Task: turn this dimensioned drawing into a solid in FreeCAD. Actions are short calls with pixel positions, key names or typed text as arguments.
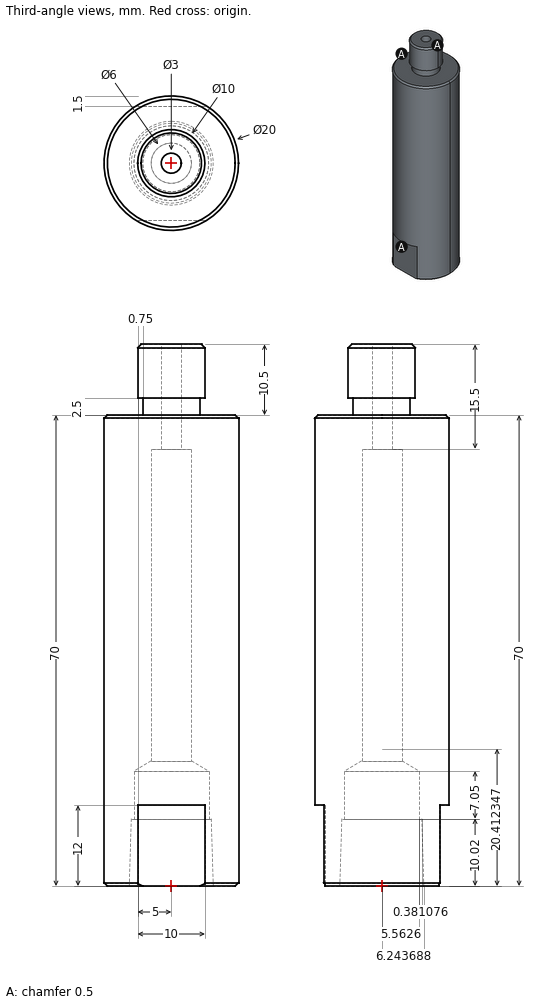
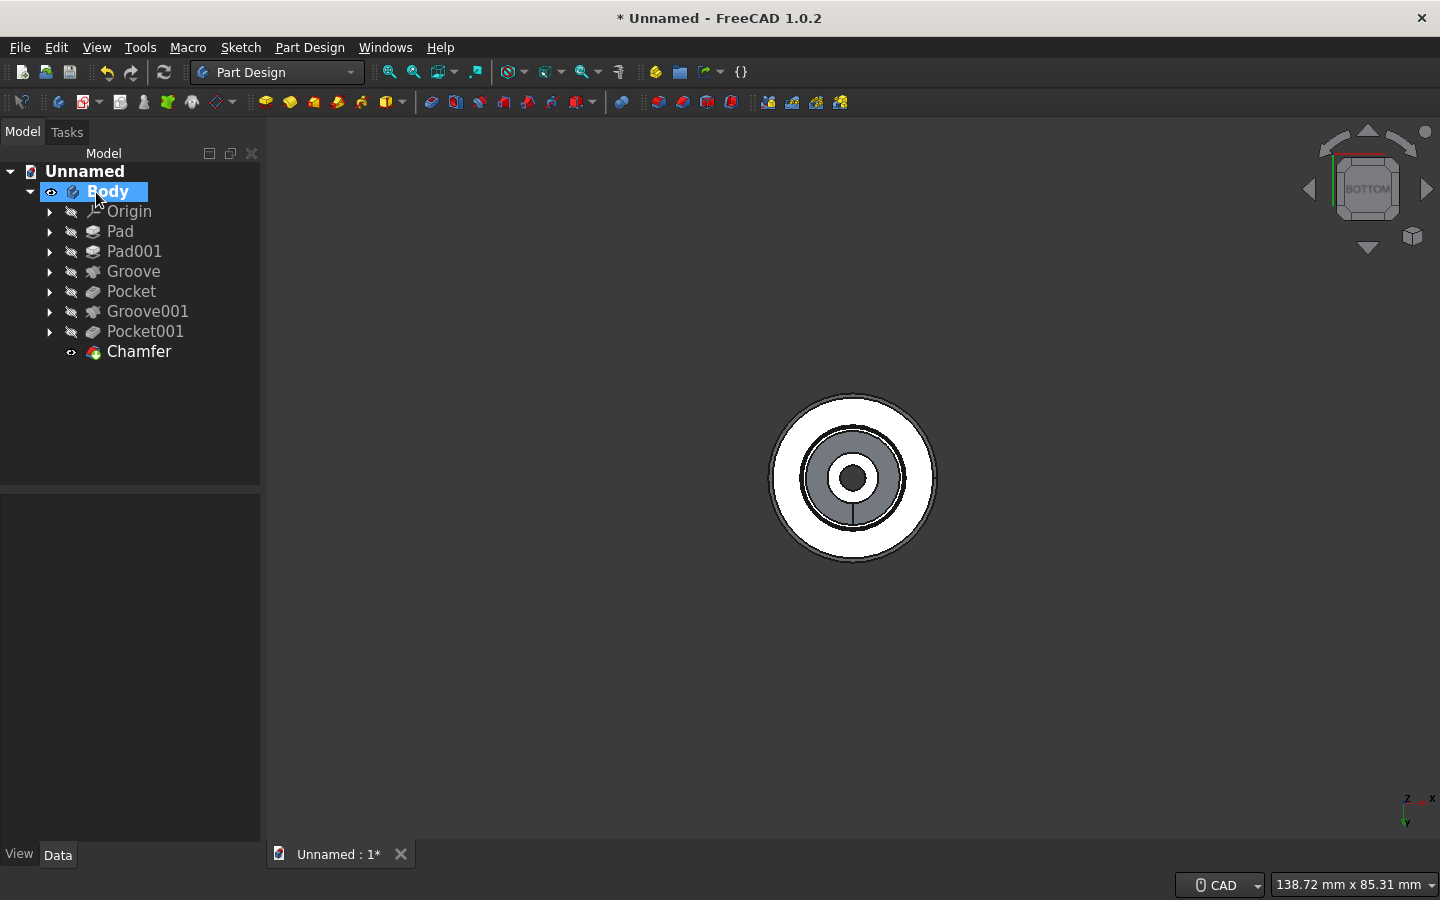
click(390, 72)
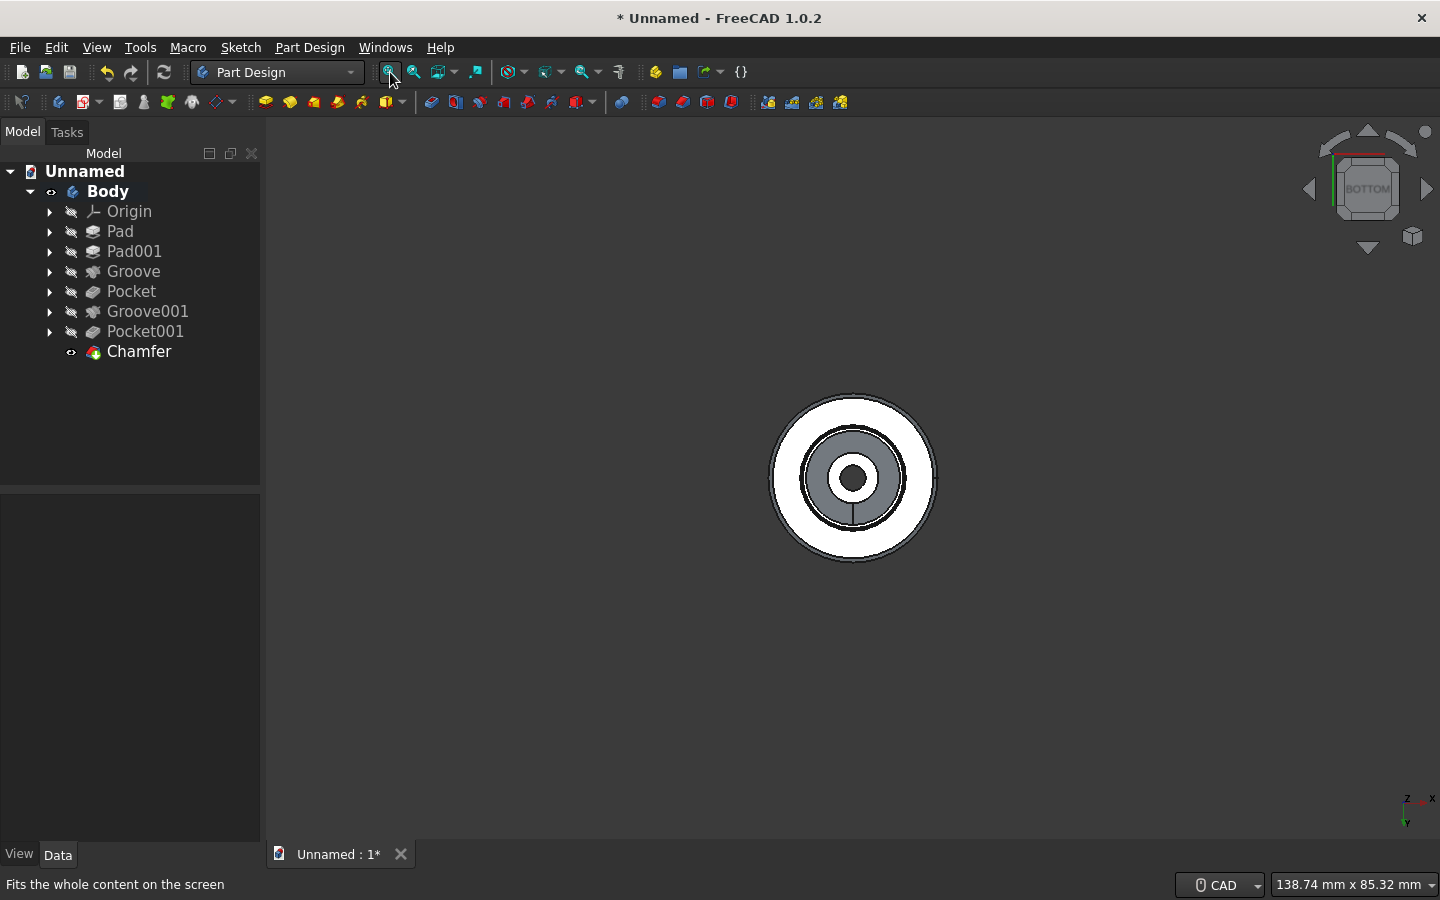
click(50, 212)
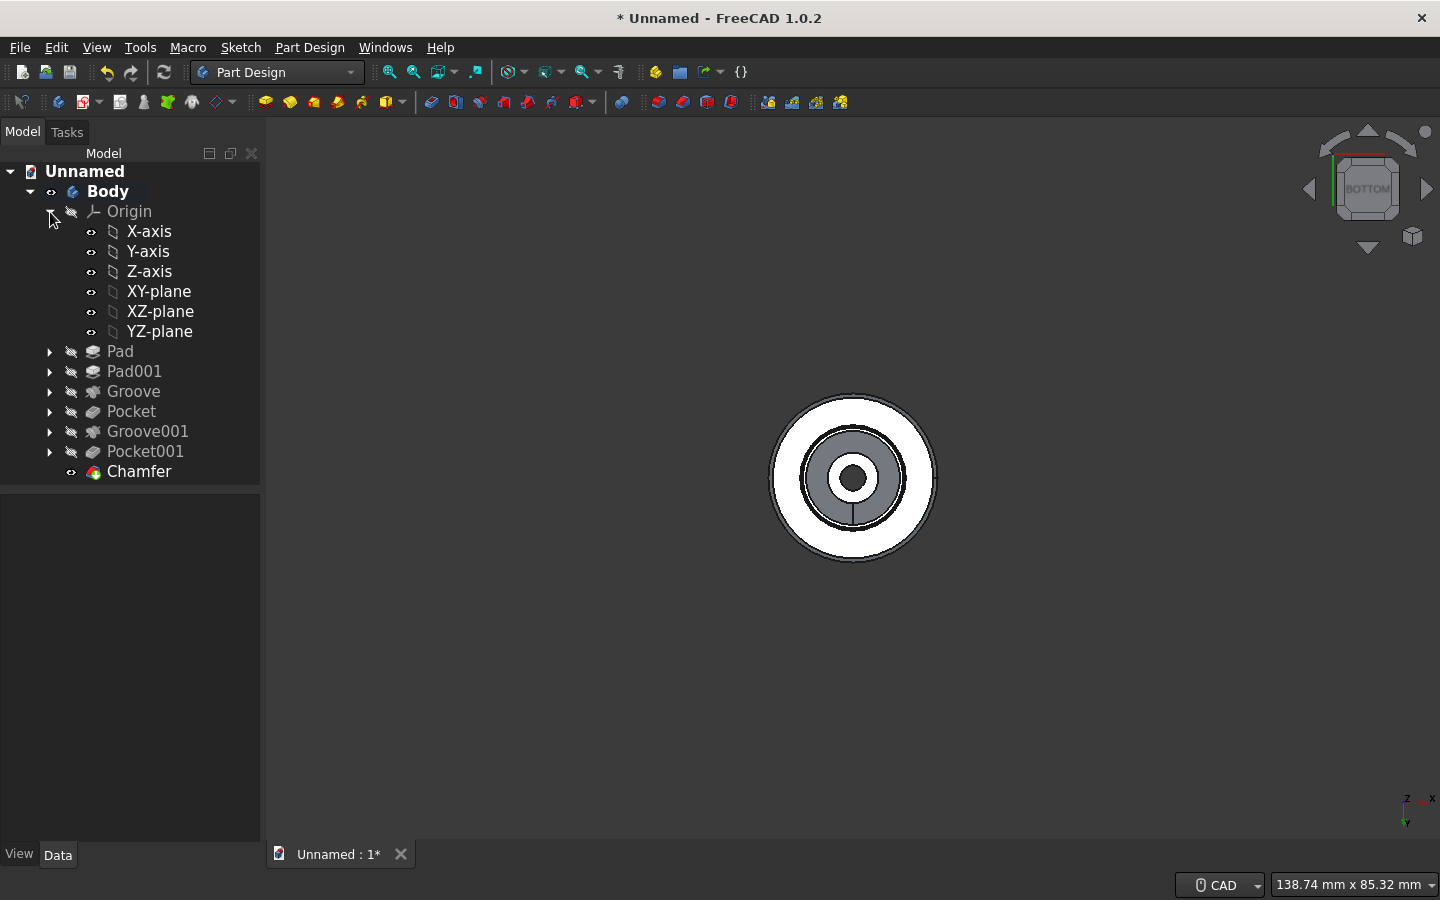
click(136, 312)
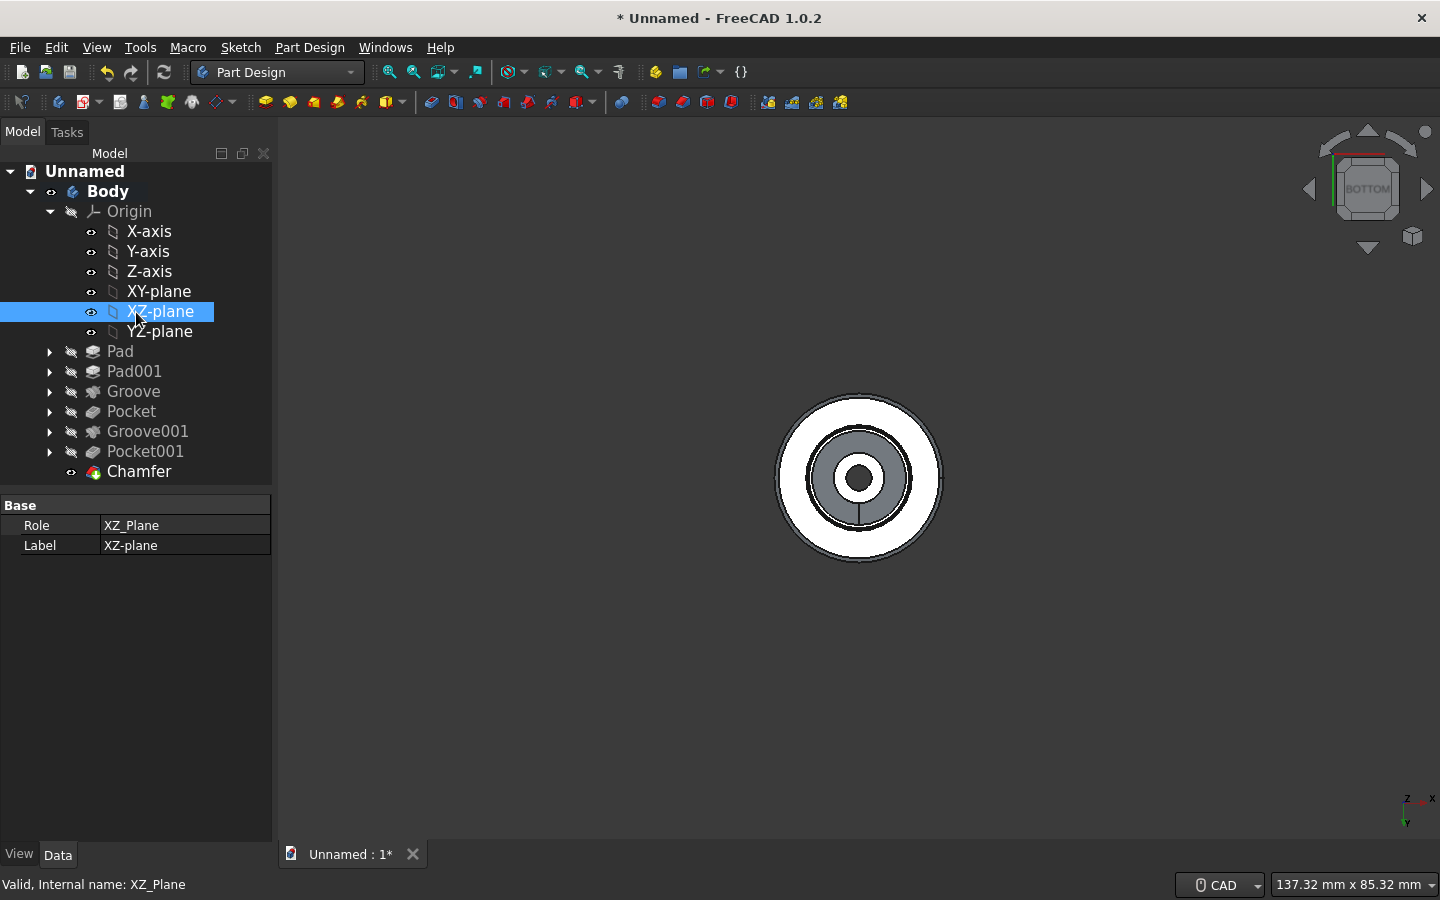
click(216, 102)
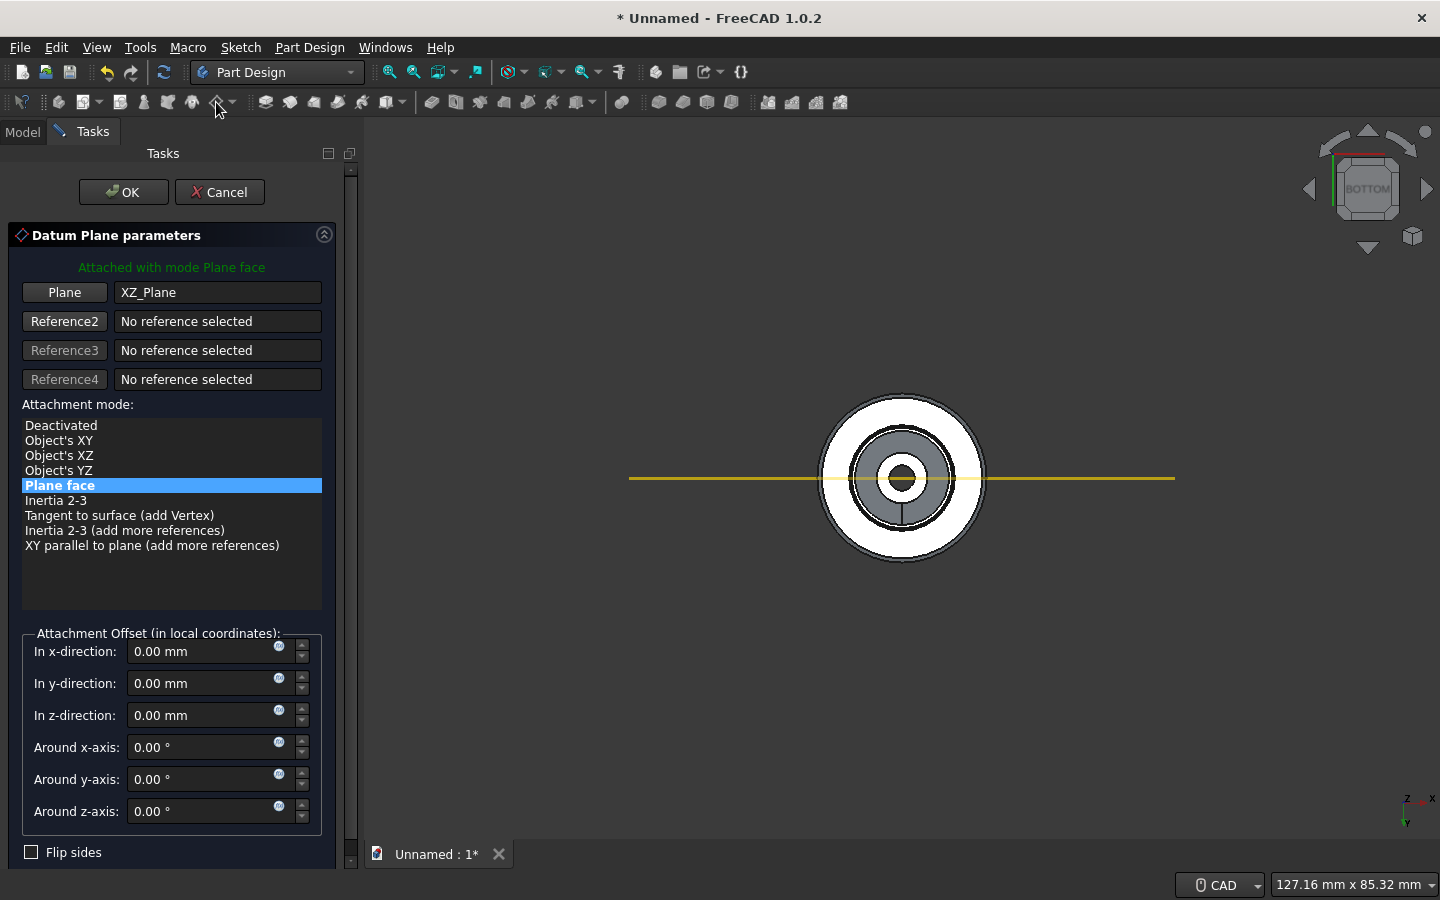
triple_click(210, 715)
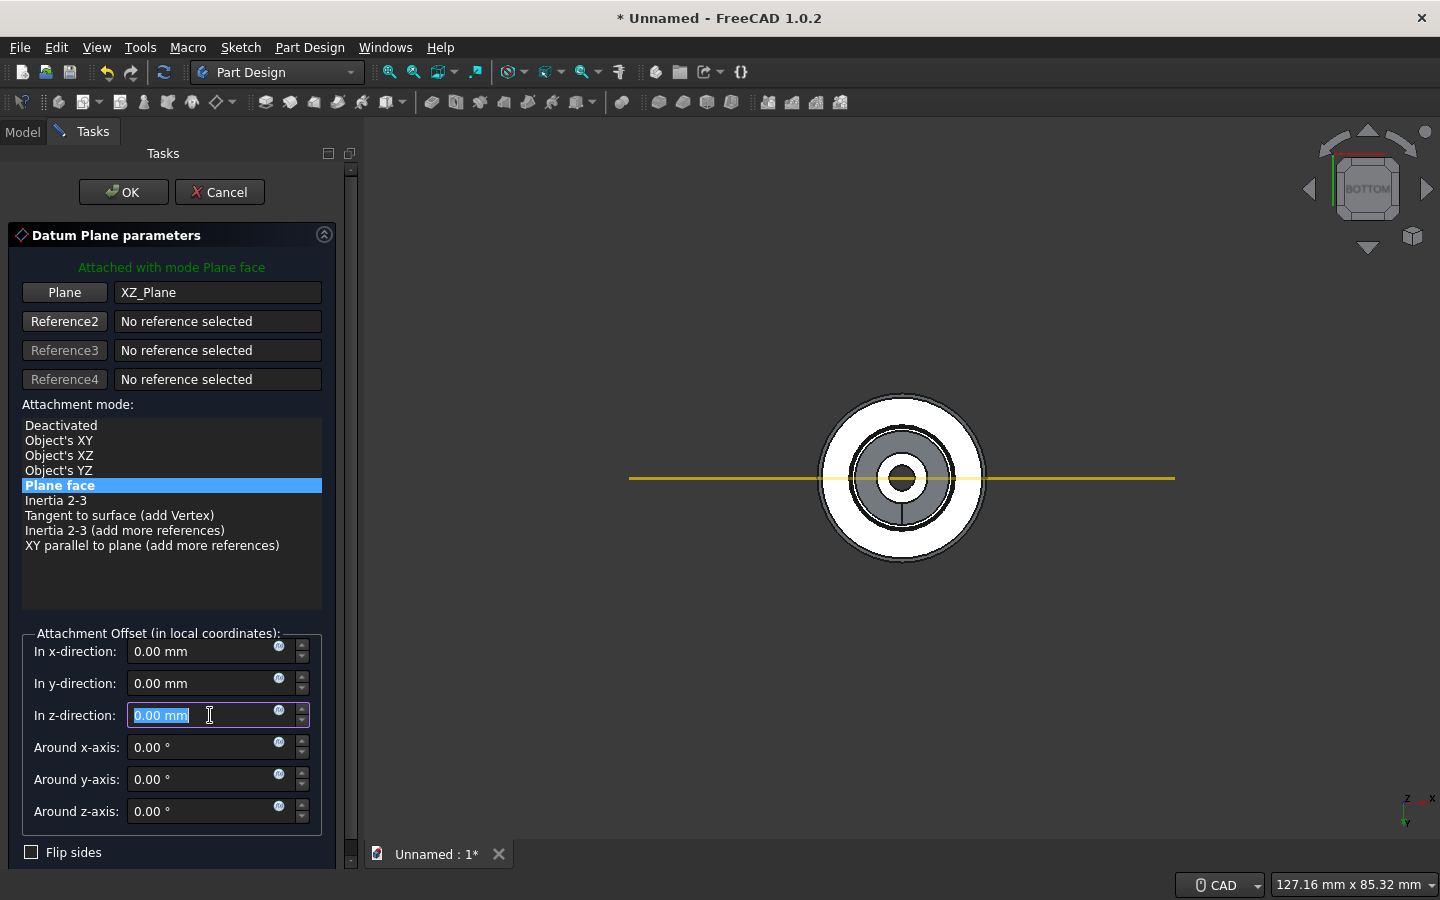
text(-10)
key(Tab)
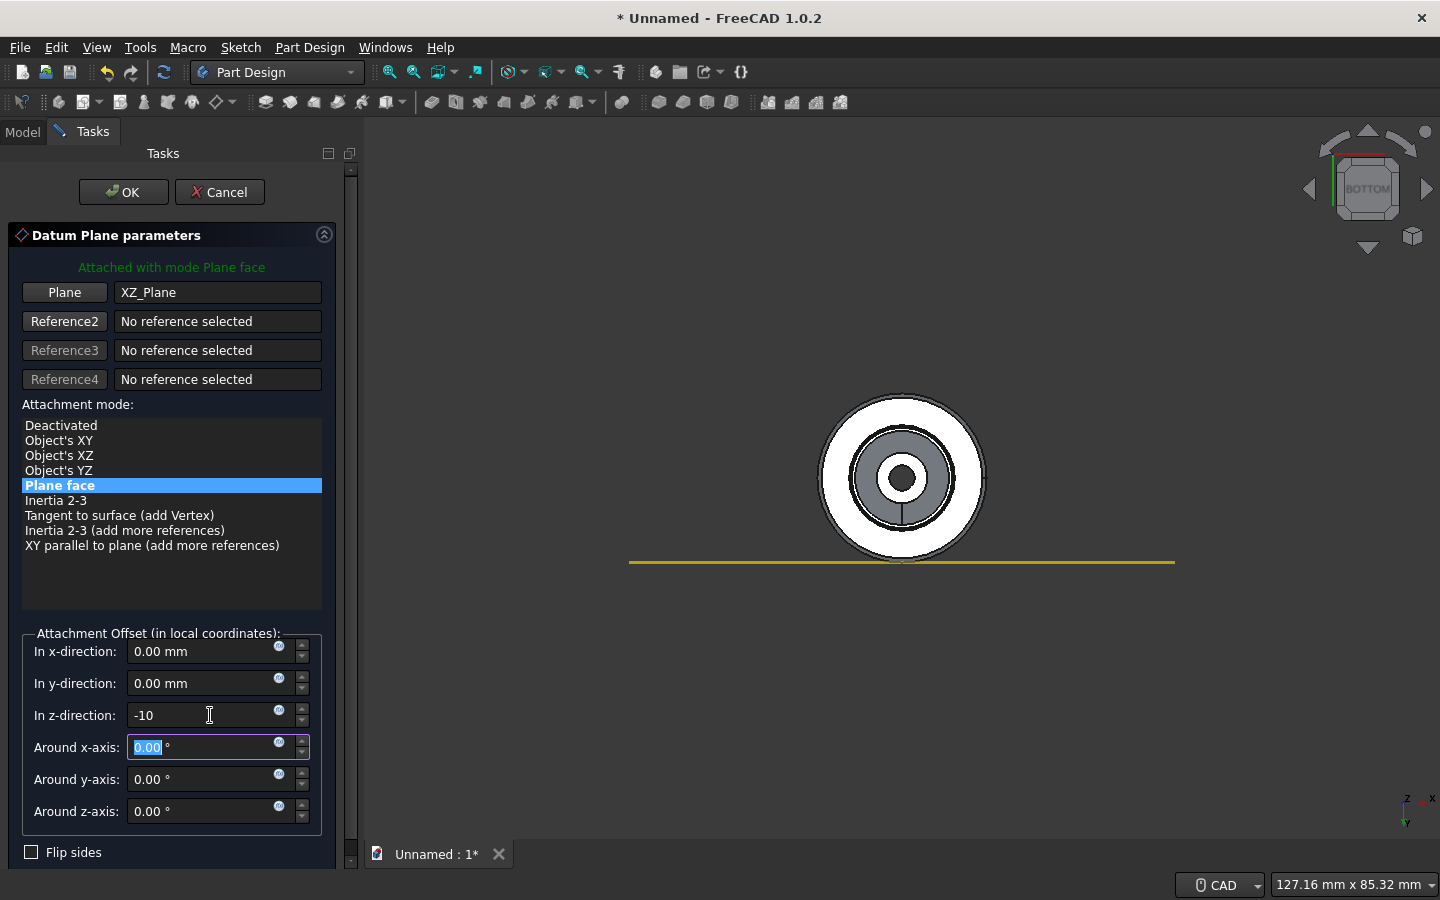
click(124, 192)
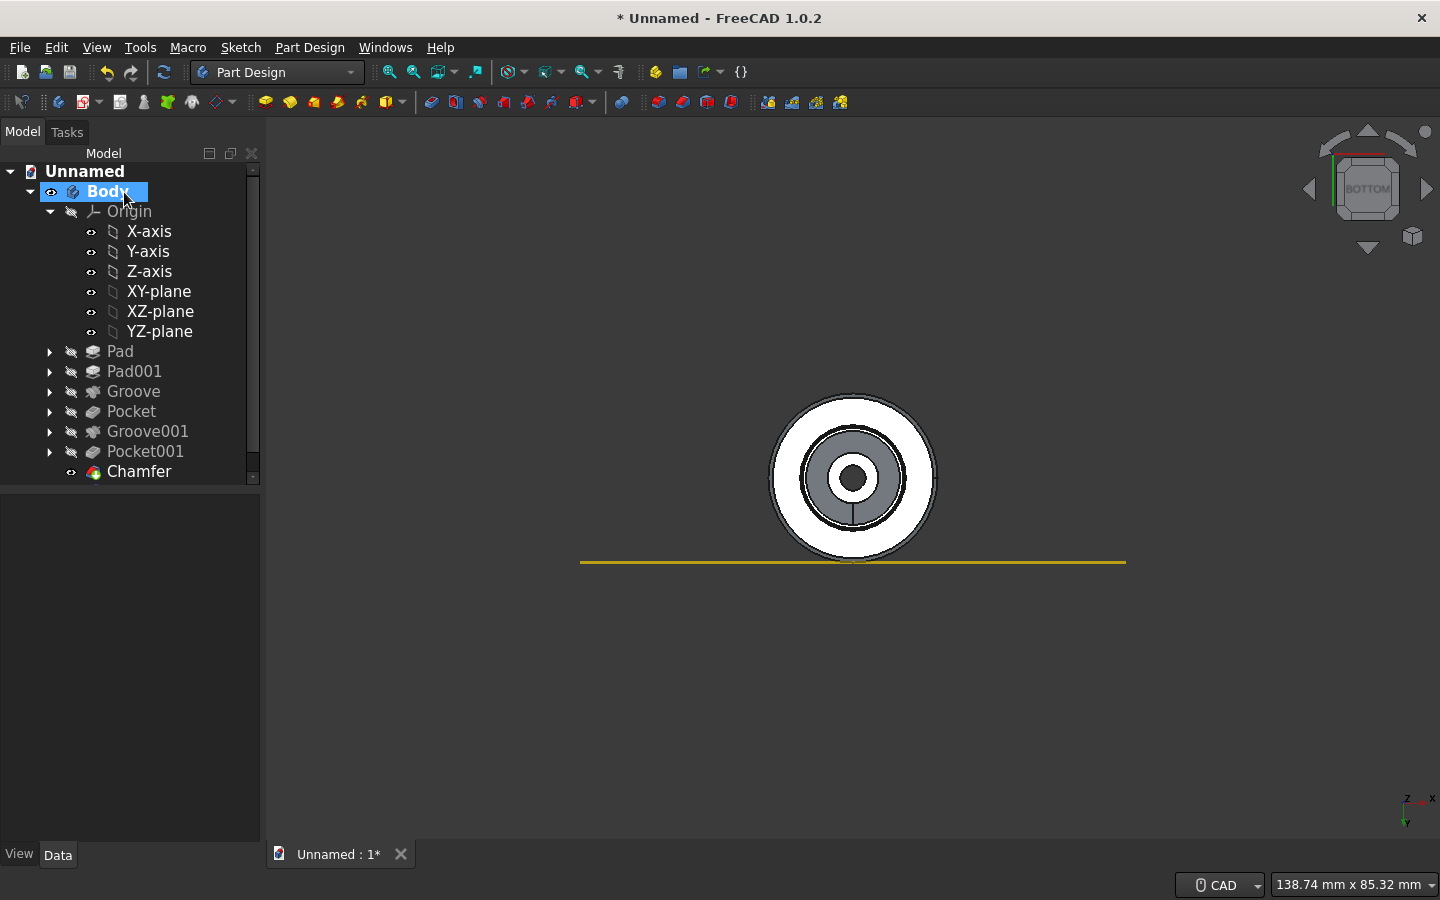
scroll(100, 327, down, 3)